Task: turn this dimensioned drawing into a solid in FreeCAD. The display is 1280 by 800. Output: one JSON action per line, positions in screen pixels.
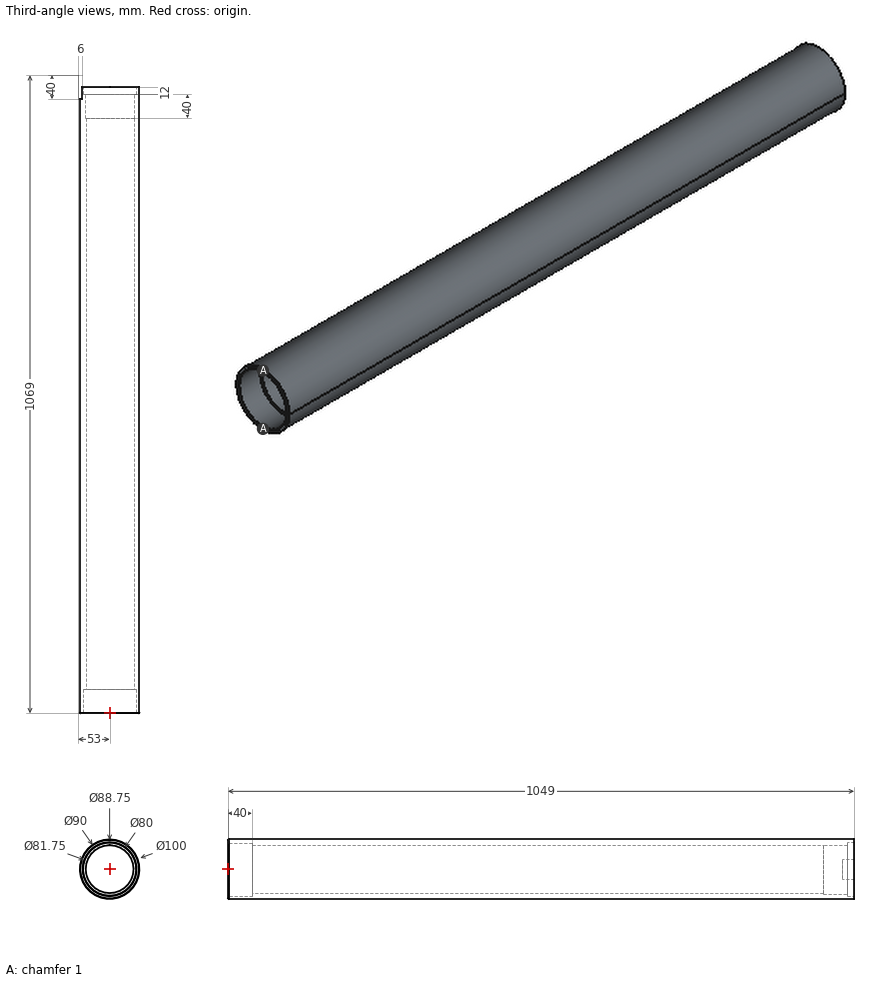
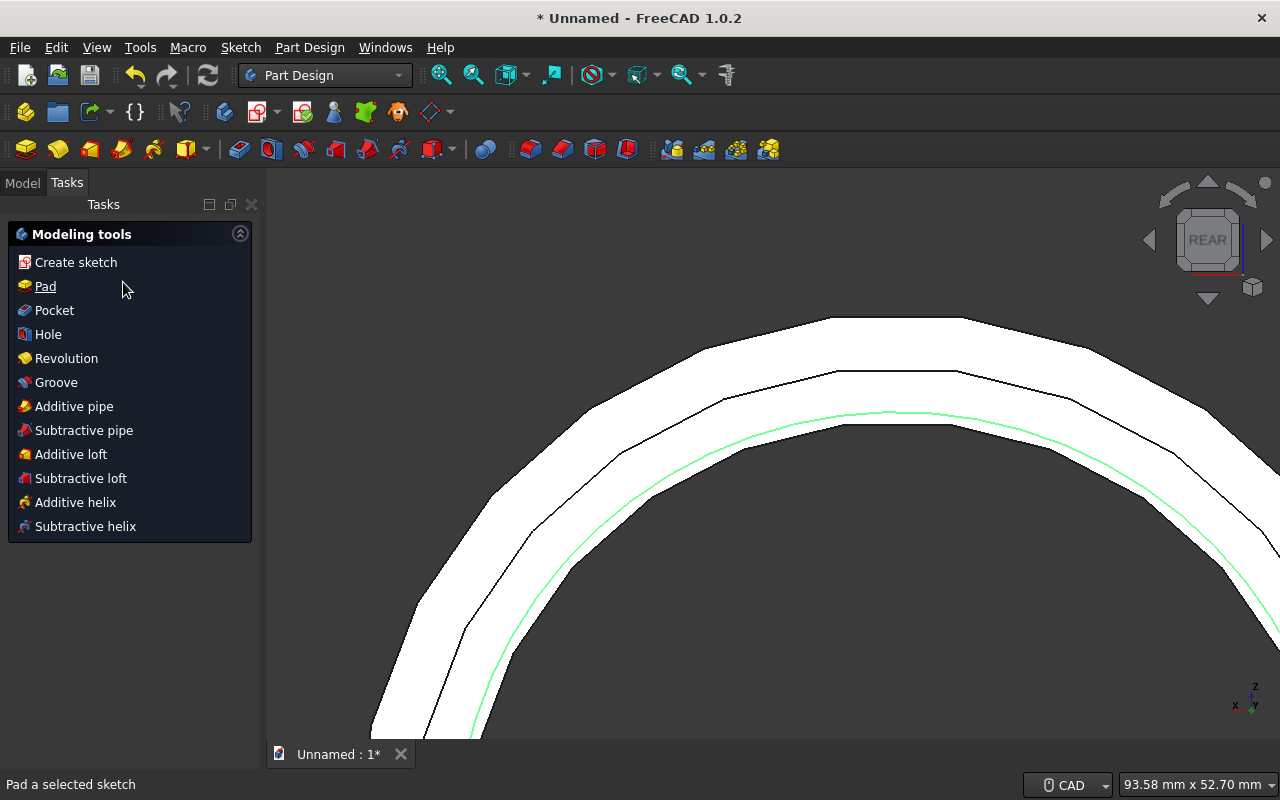
{"action": "left_click", "coordinate": [240, 150]}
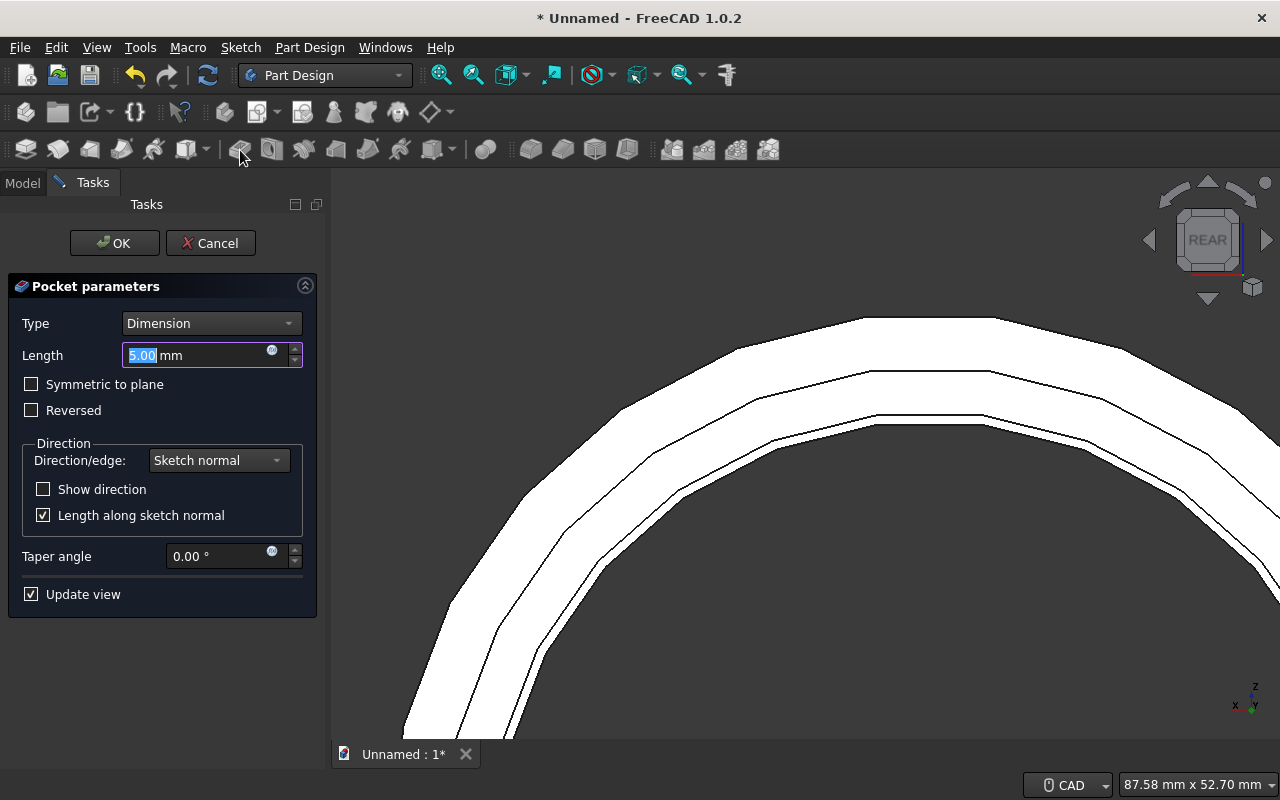
{"action": "type", "text": "40"}
{"action": "key", "text": "Tab"}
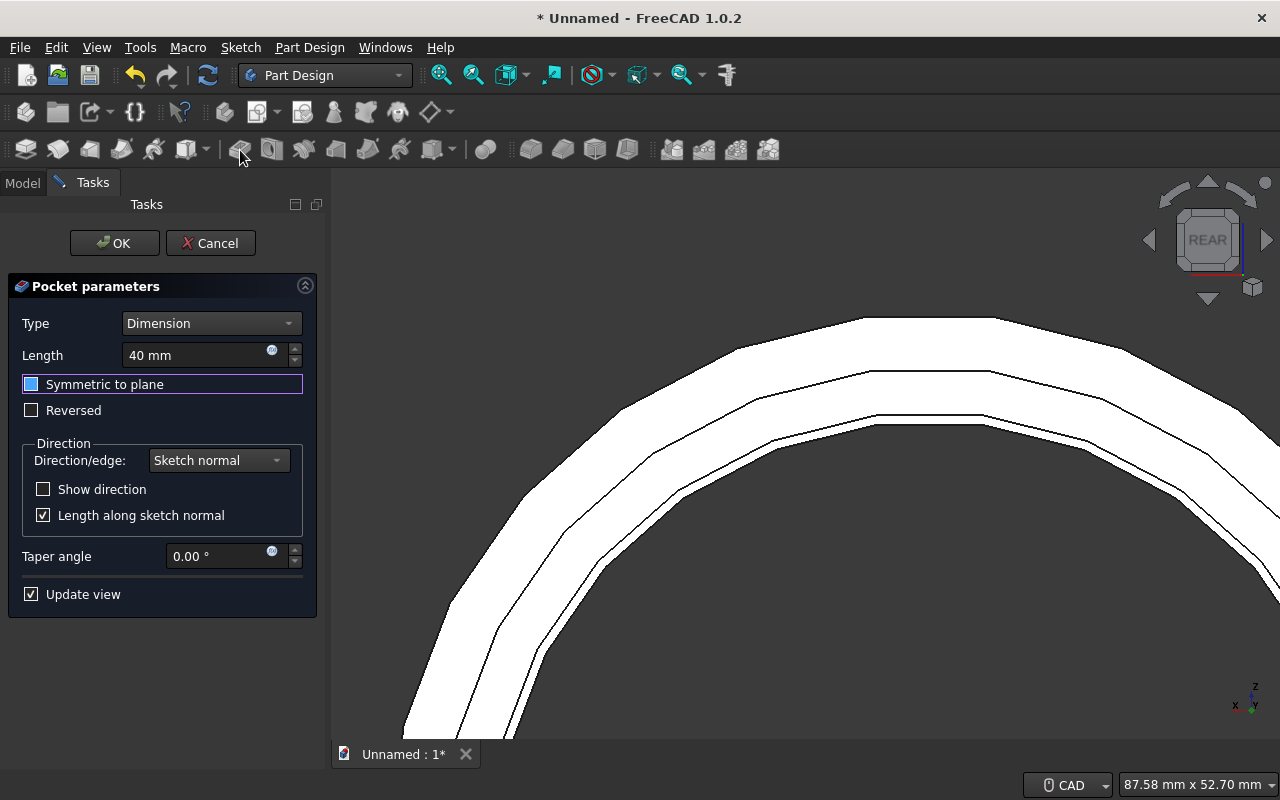
{"action": "left_click", "coordinate": [115, 243]}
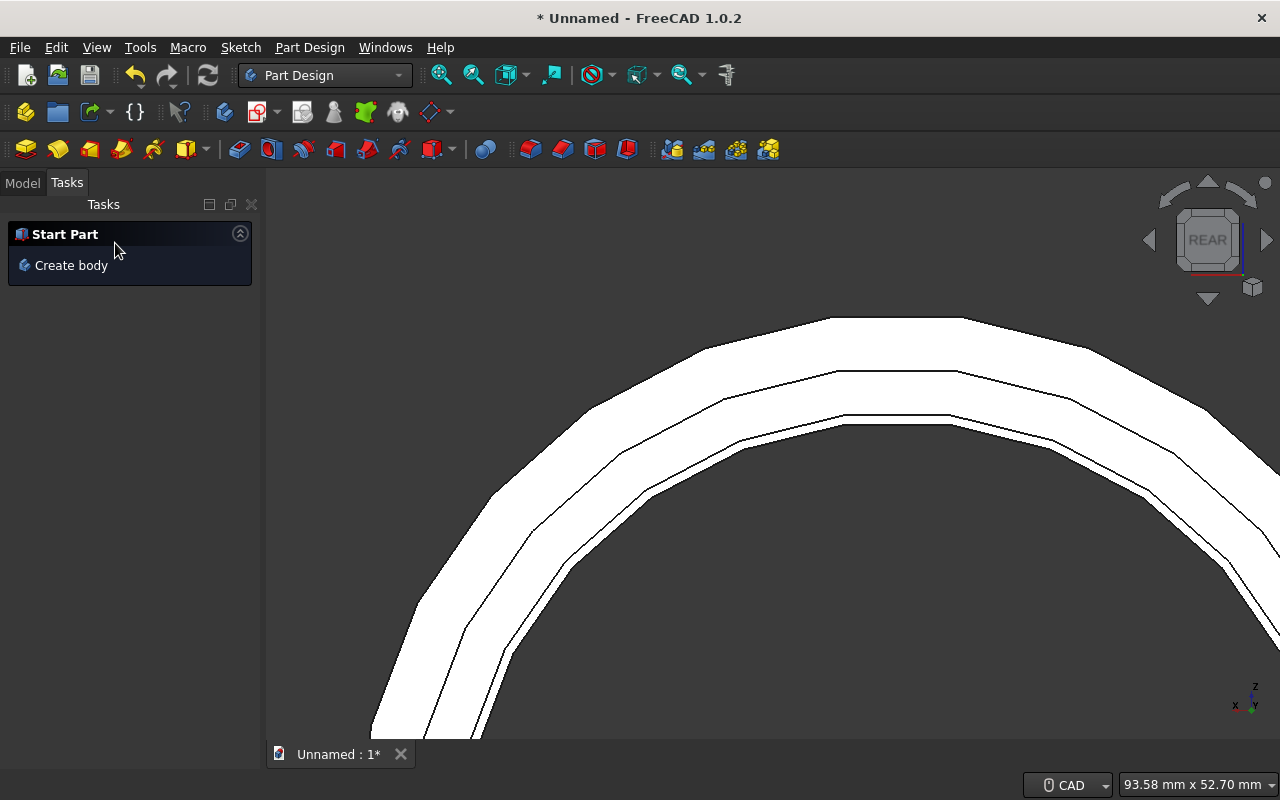
{"action": "left_click", "coordinate": [442, 76]}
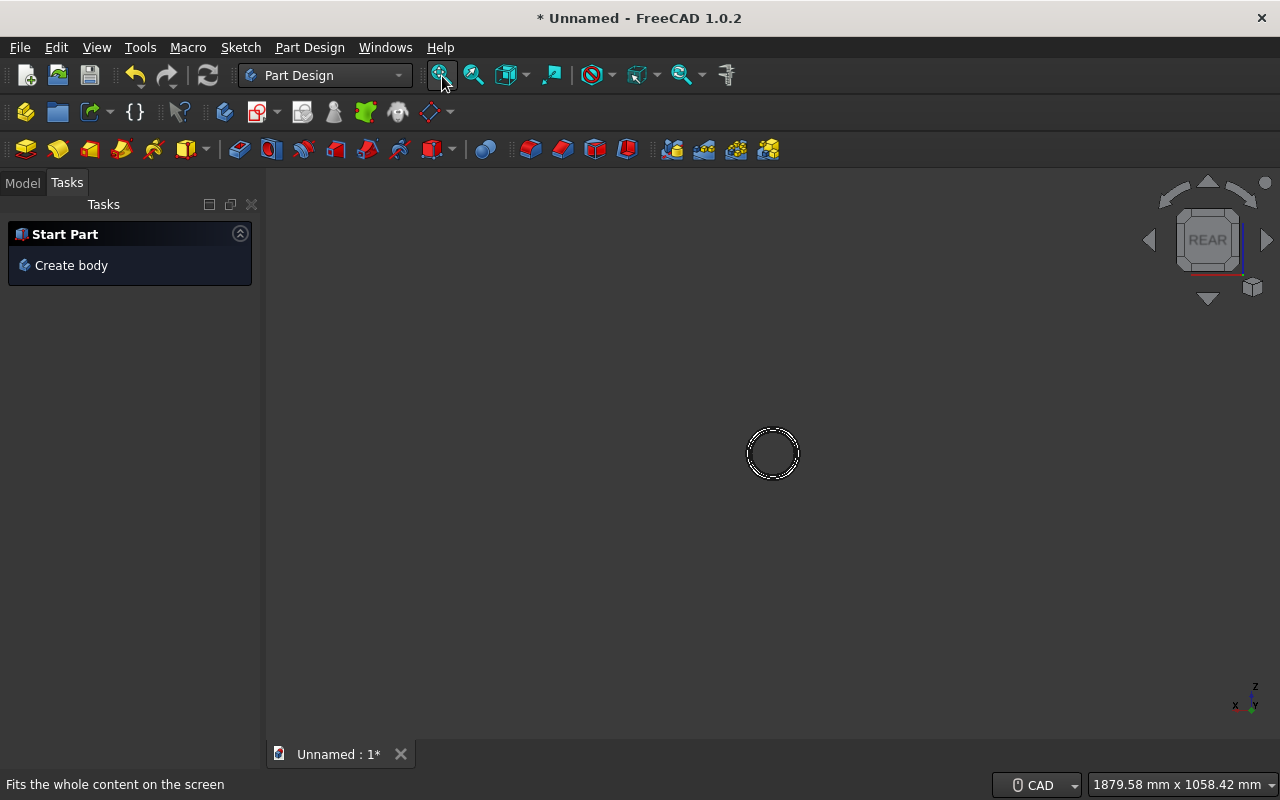
{"action": "left_click", "coordinate": [258, 112]}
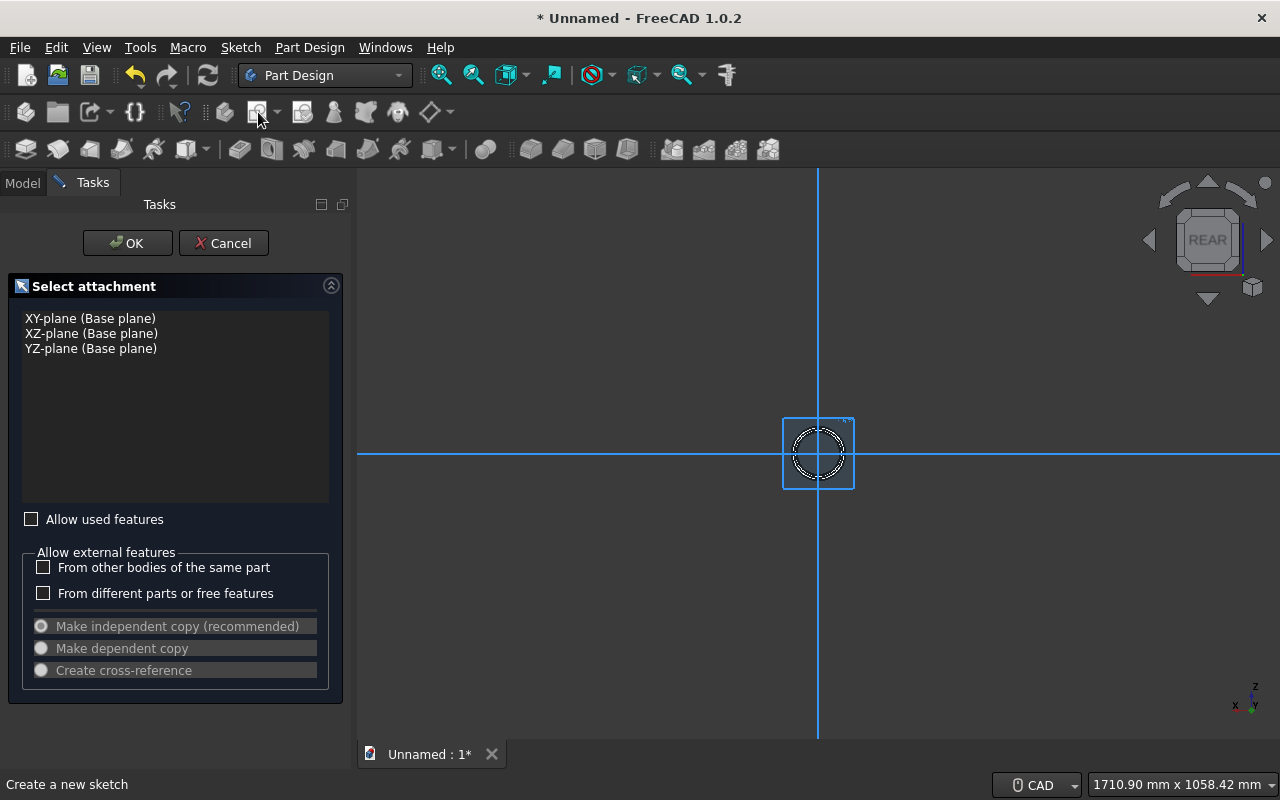
{"action": "left_click", "coordinate": [82, 318]}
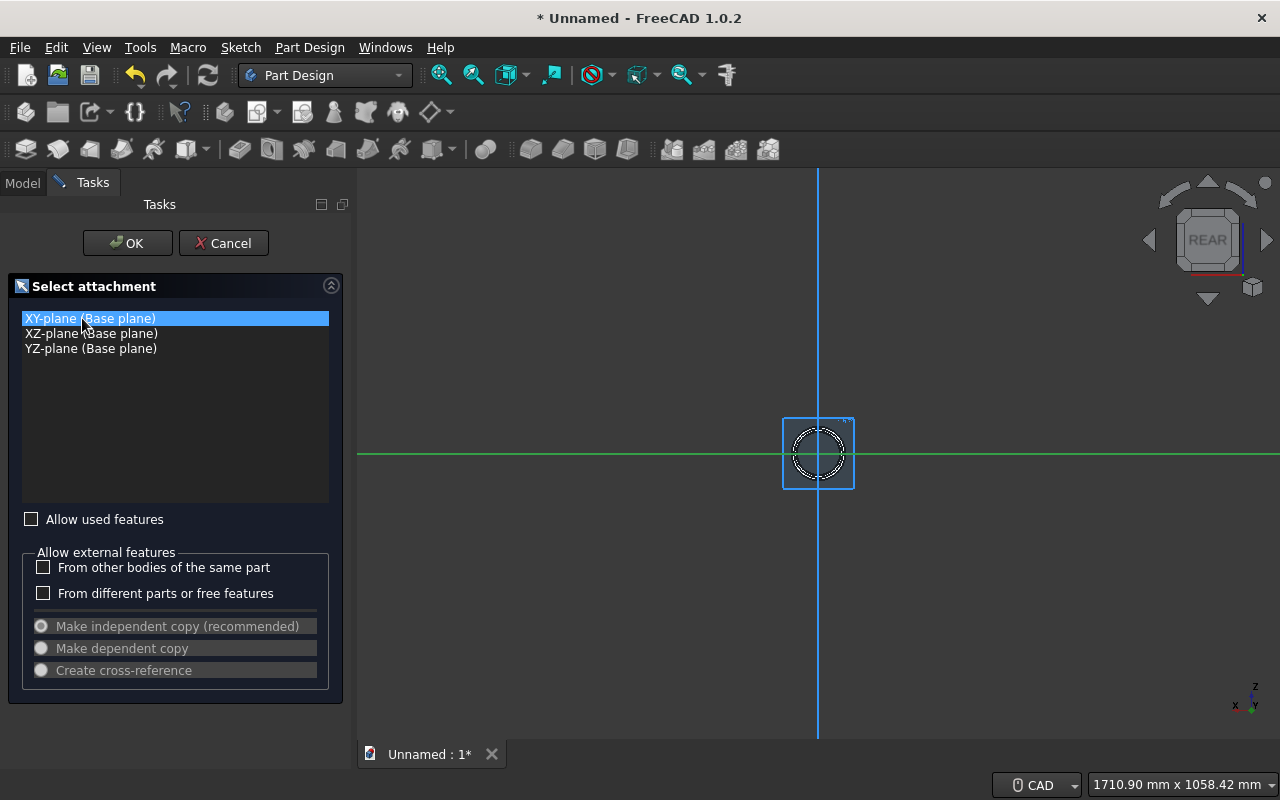
{"action": "left_click", "coordinate": [128, 243]}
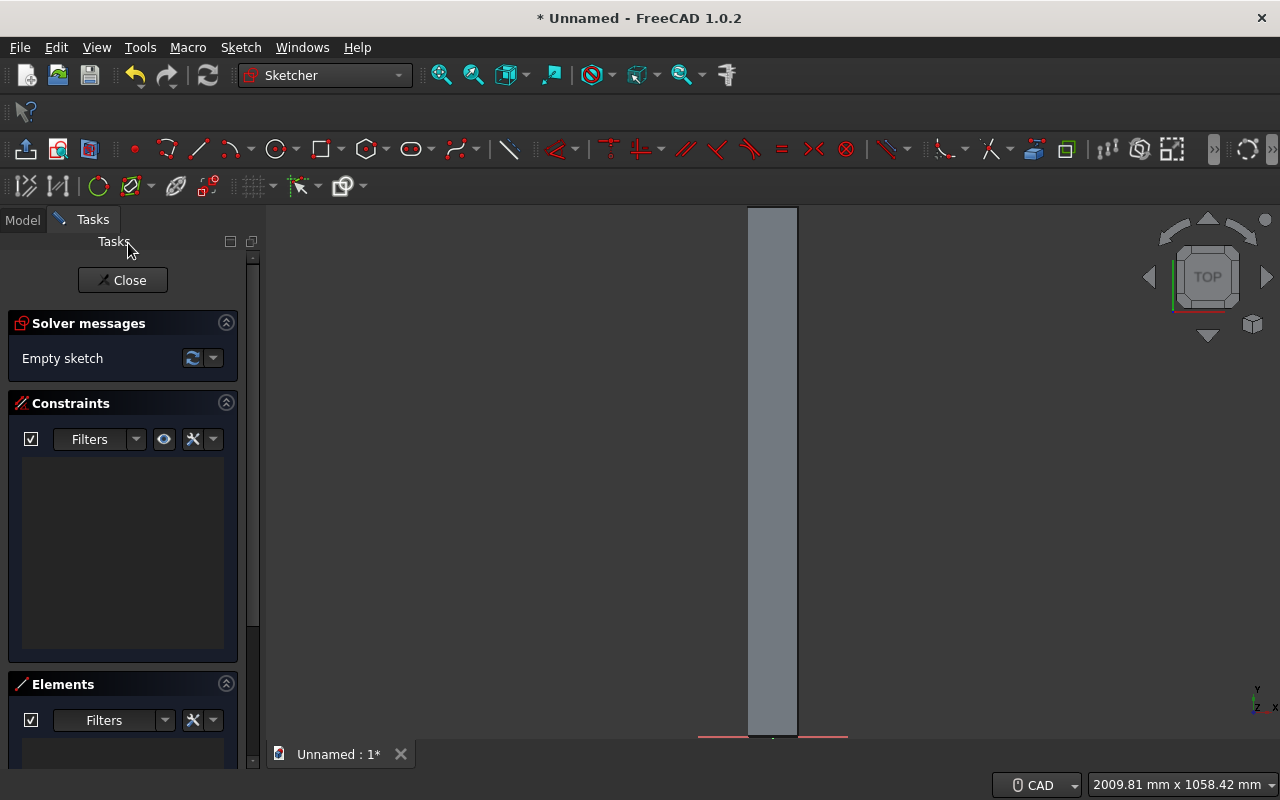
{"action": "left_click", "coordinate": [90, 150]}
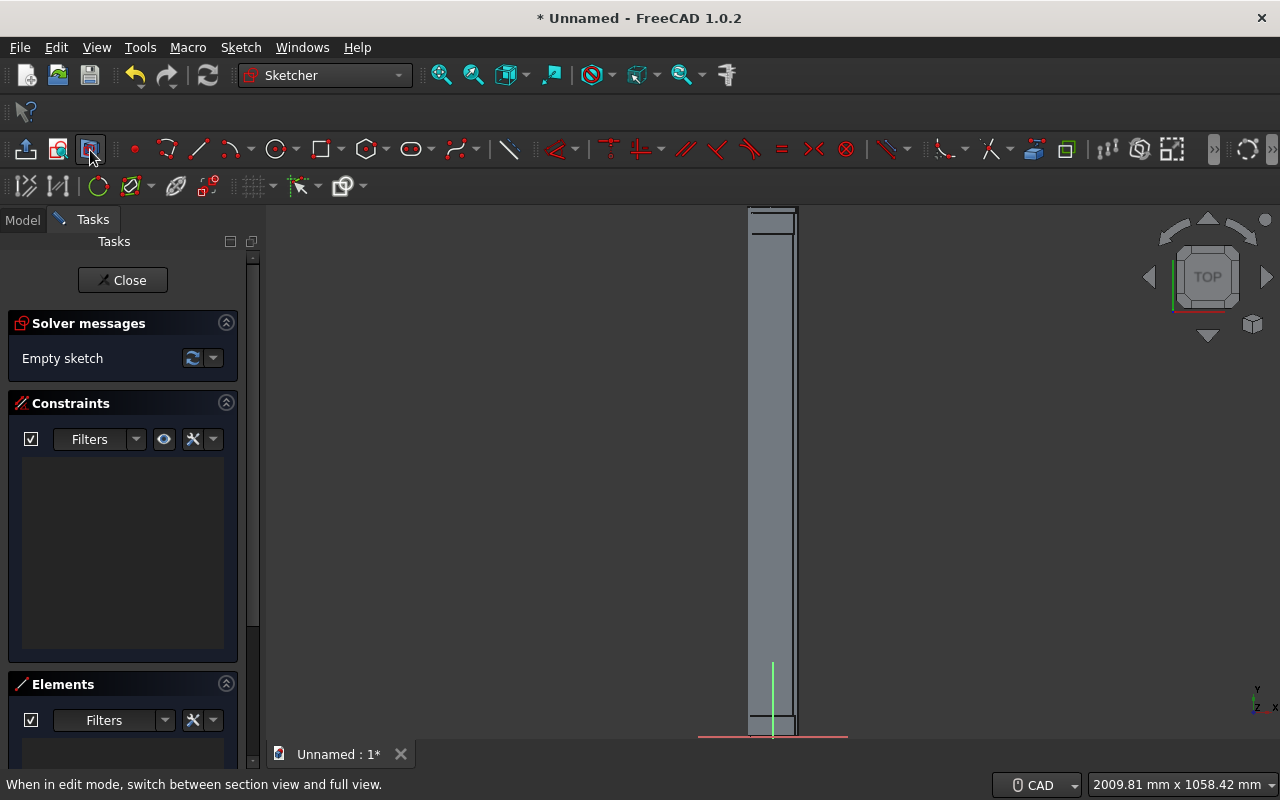
{"action": "scroll", "coordinate": [704, 472], "scroll_direction": "down", "scroll_amount": 5}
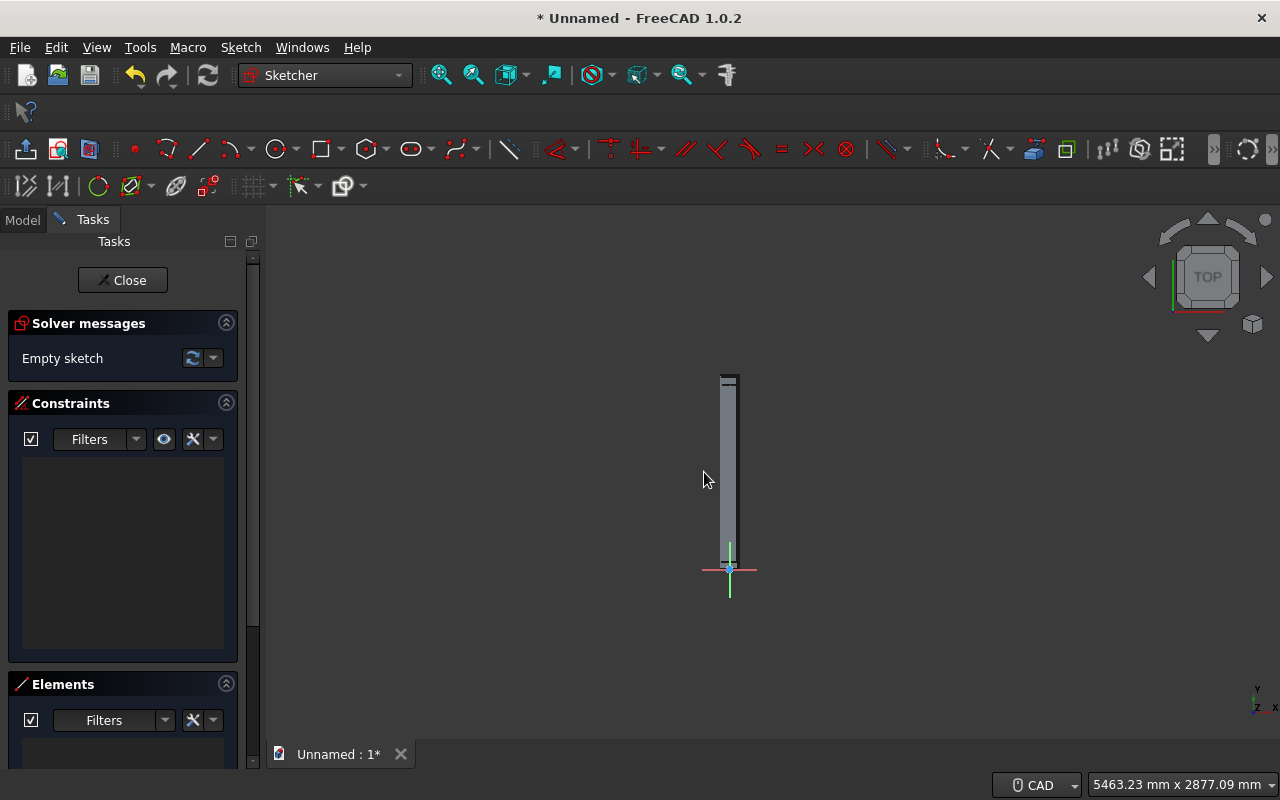
{"action": "scroll", "coordinate": [721, 370], "scroll_direction": "up", "scroll_amount": 15}